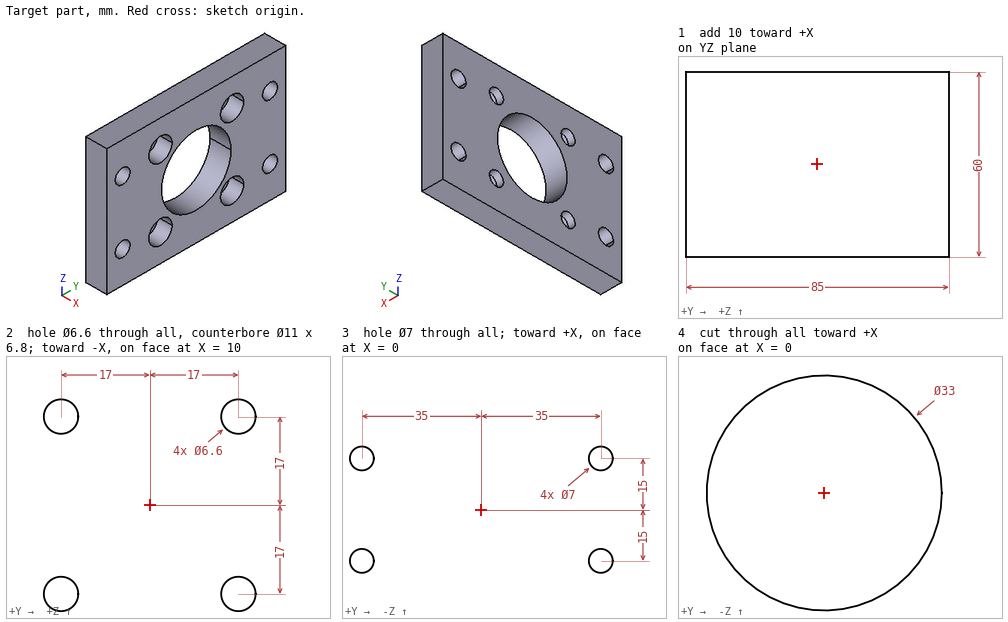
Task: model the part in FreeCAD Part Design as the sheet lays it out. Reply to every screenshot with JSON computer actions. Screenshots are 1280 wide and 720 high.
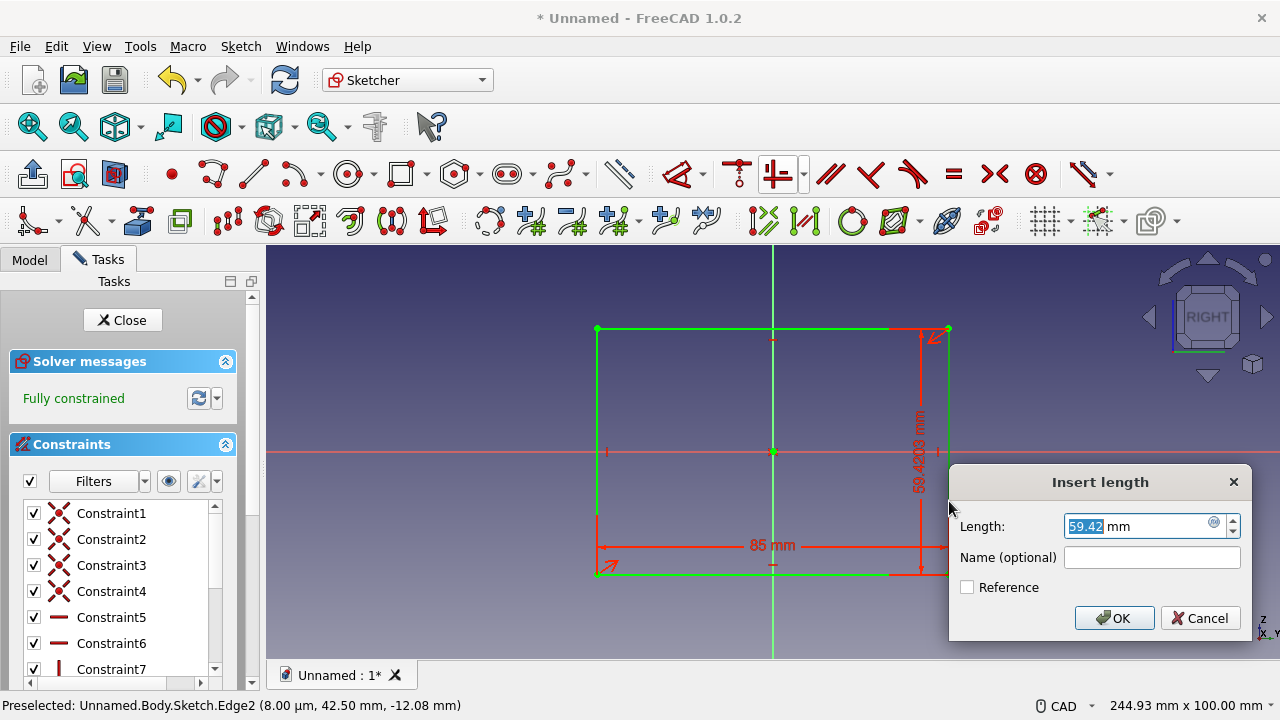
{"action": "type", "text": "60"}
{"action": "key", "text": "Return"}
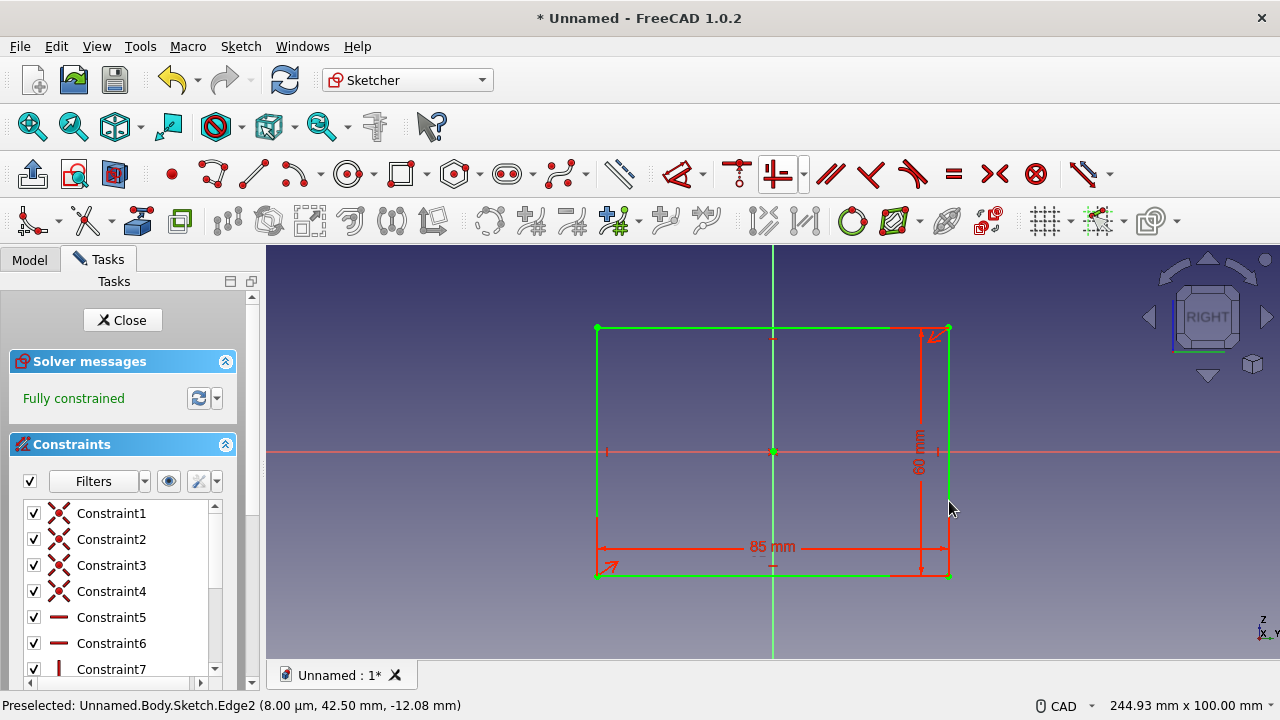
{"action": "left_click", "coordinate": [123, 320]}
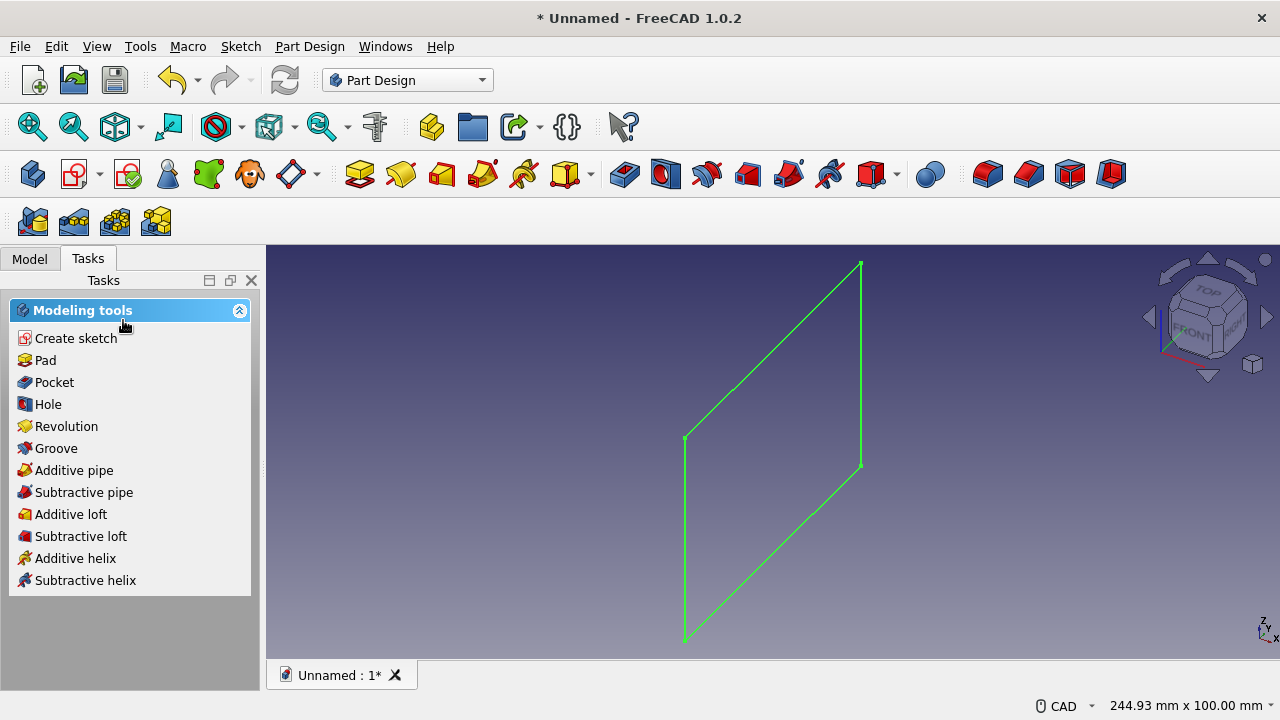
{"action": "left_click", "coordinate": [360, 174]}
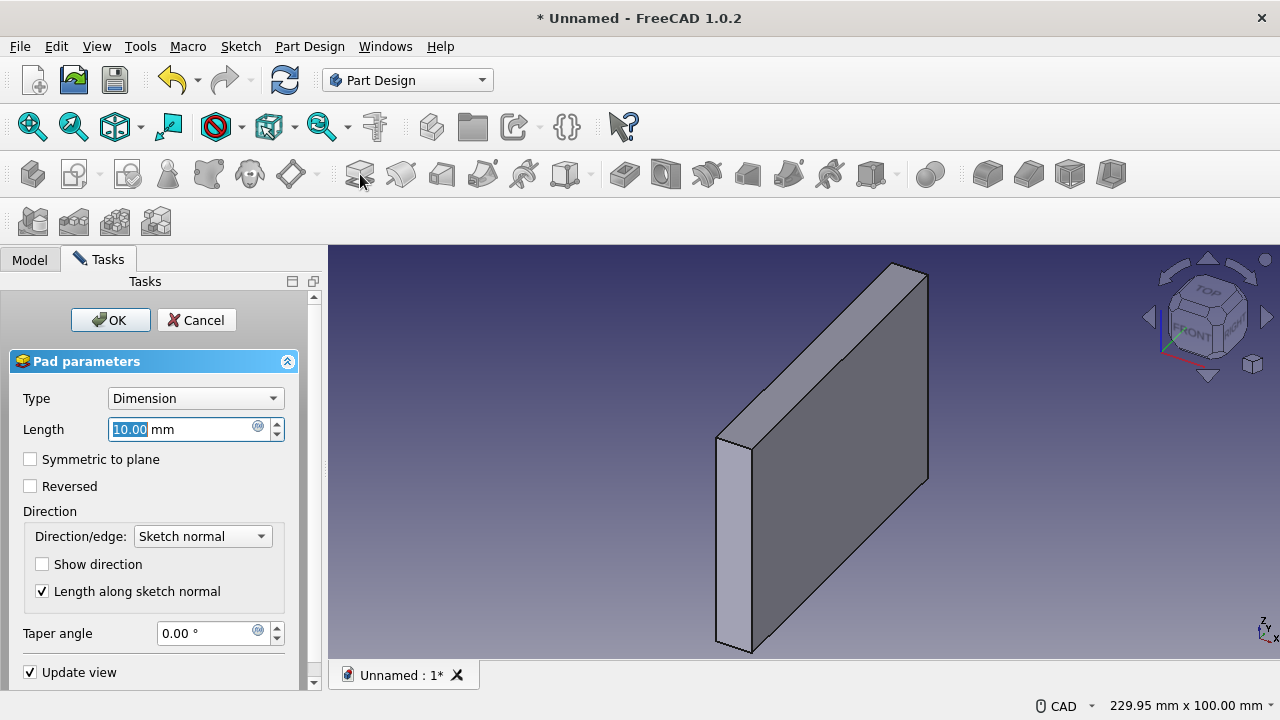
{"action": "type", "text": "10"}
{"action": "key", "text": "Tab"}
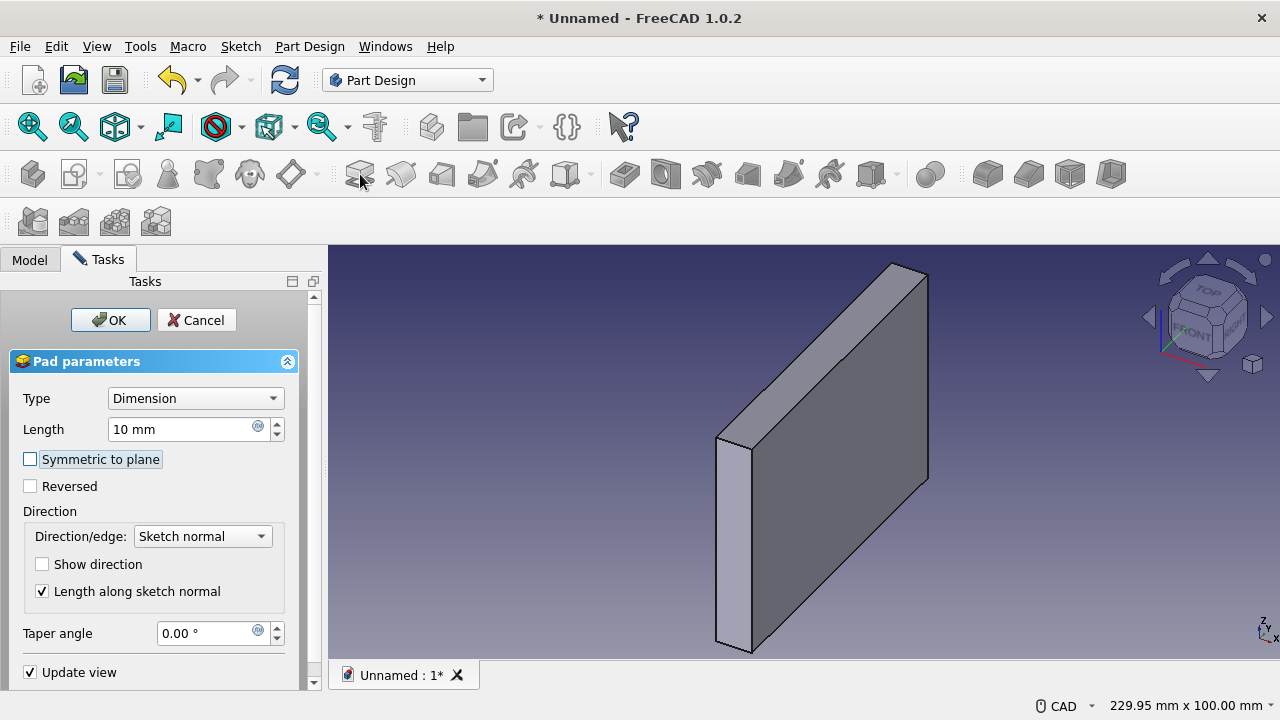
{"action": "left_click", "coordinate": [111, 320]}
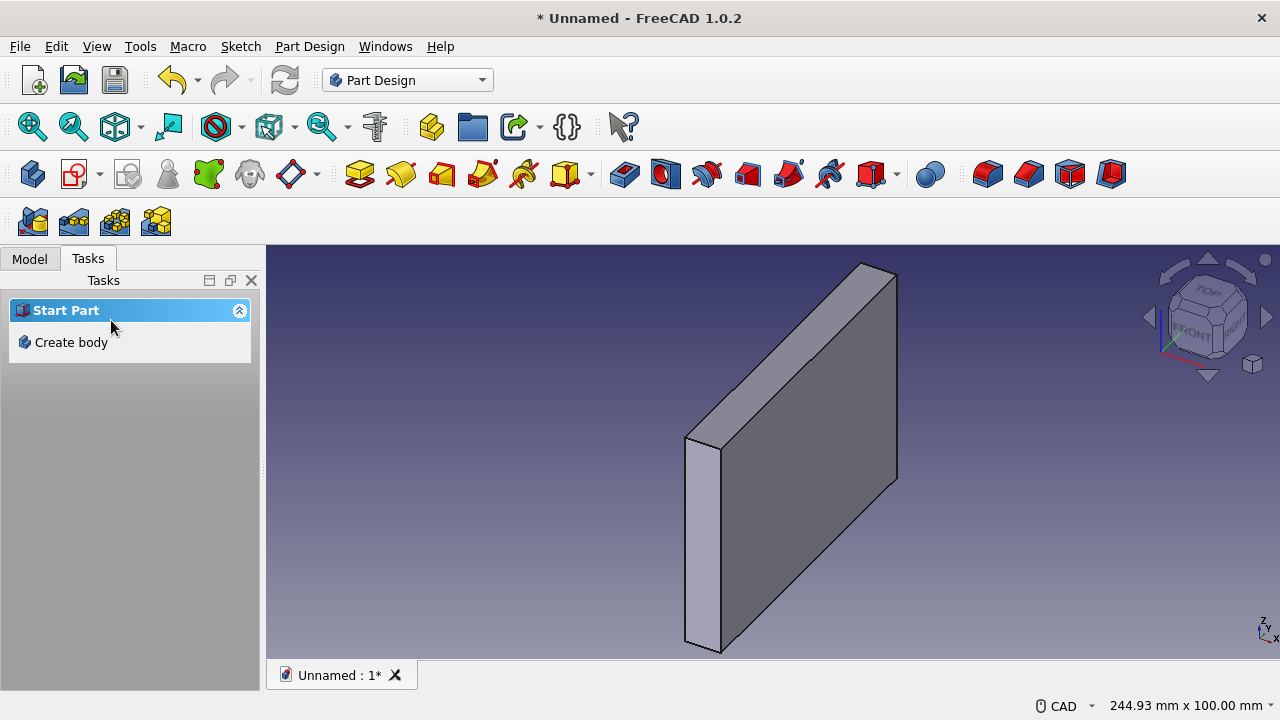
{"action": "left_click", "coordinate": [834, 438]}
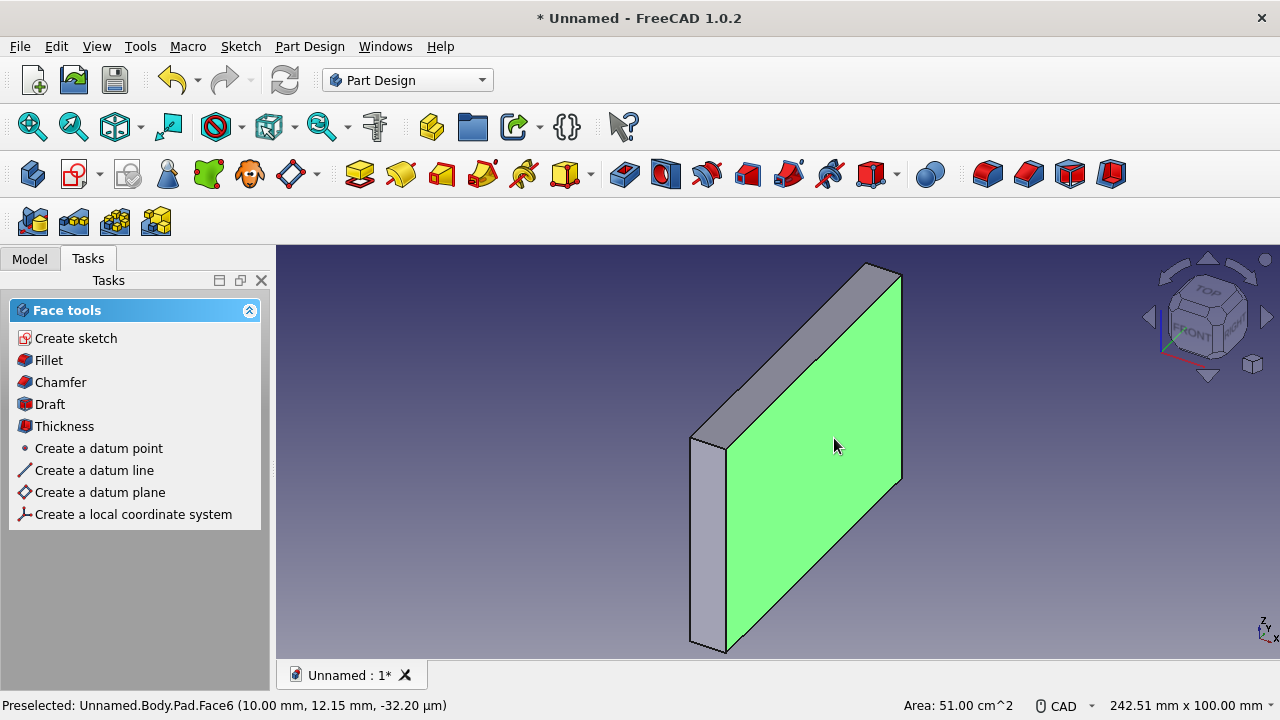
{"action": "left_click", "coordinate": [74, 174]}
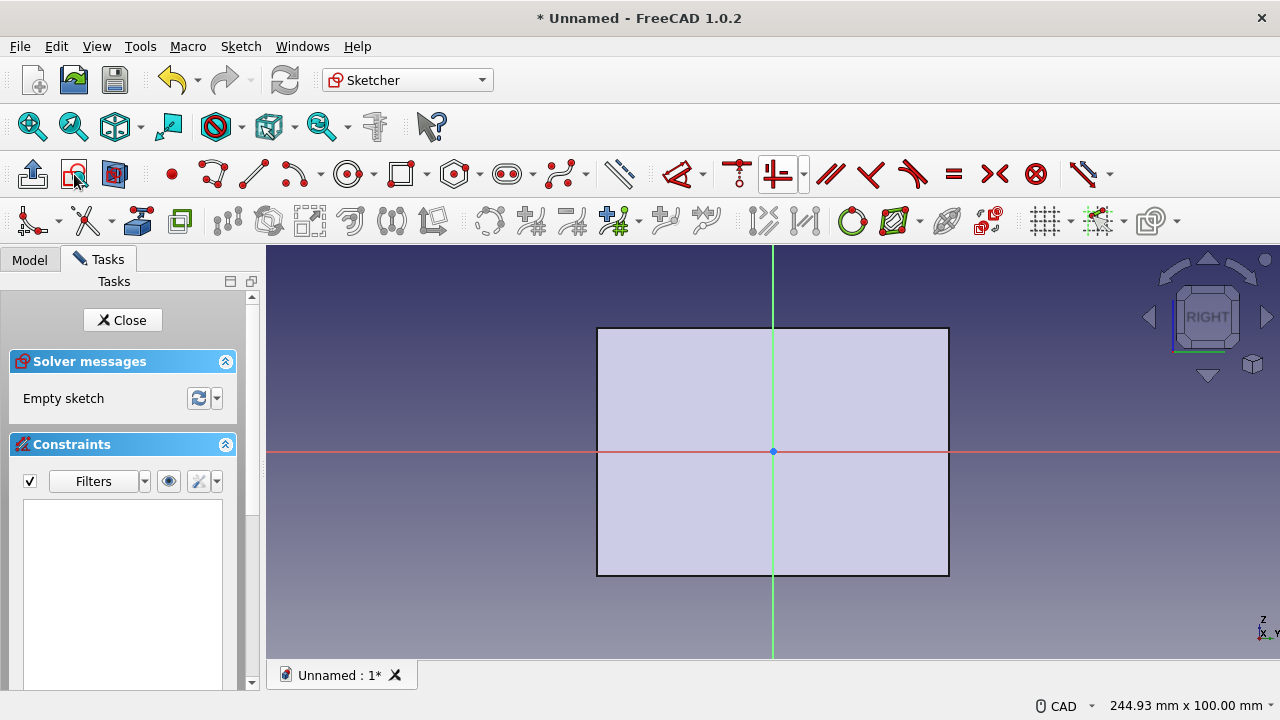
{"action": "scroll", "coordinate": [912, 452], "scroll_direction": "up", "scroll_amount": 2}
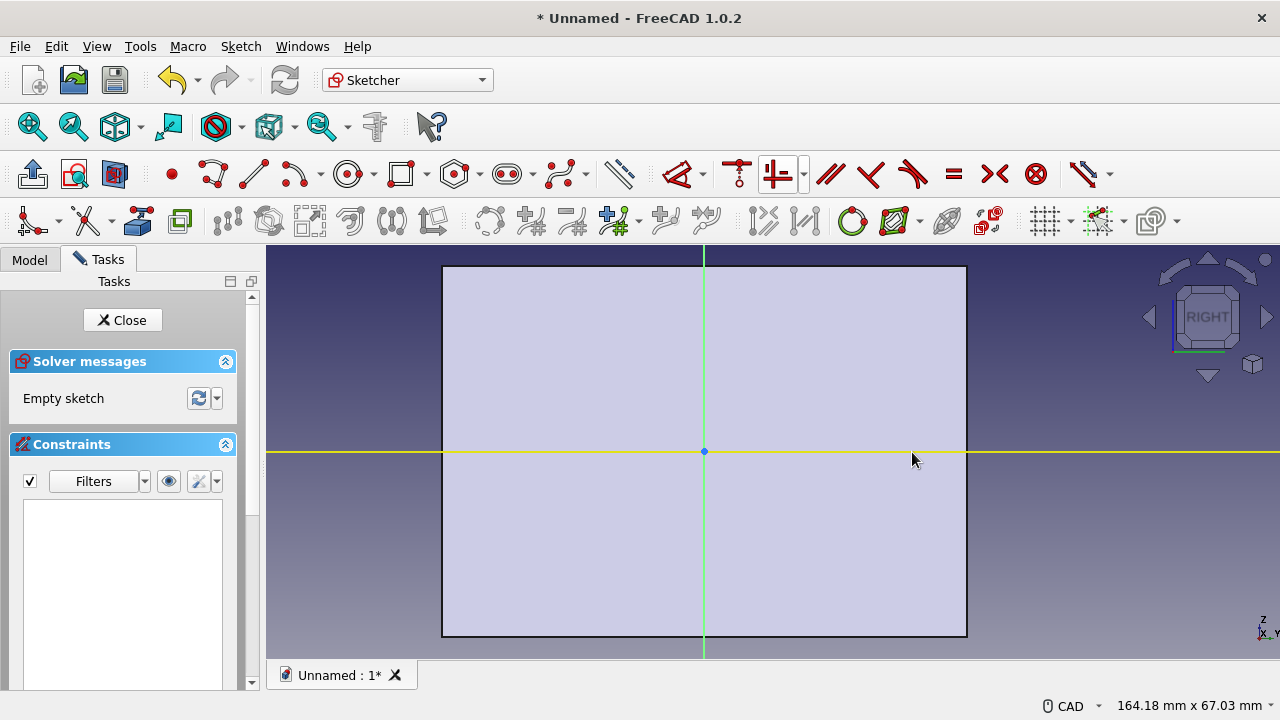
{"action": "key", "text": "g c"}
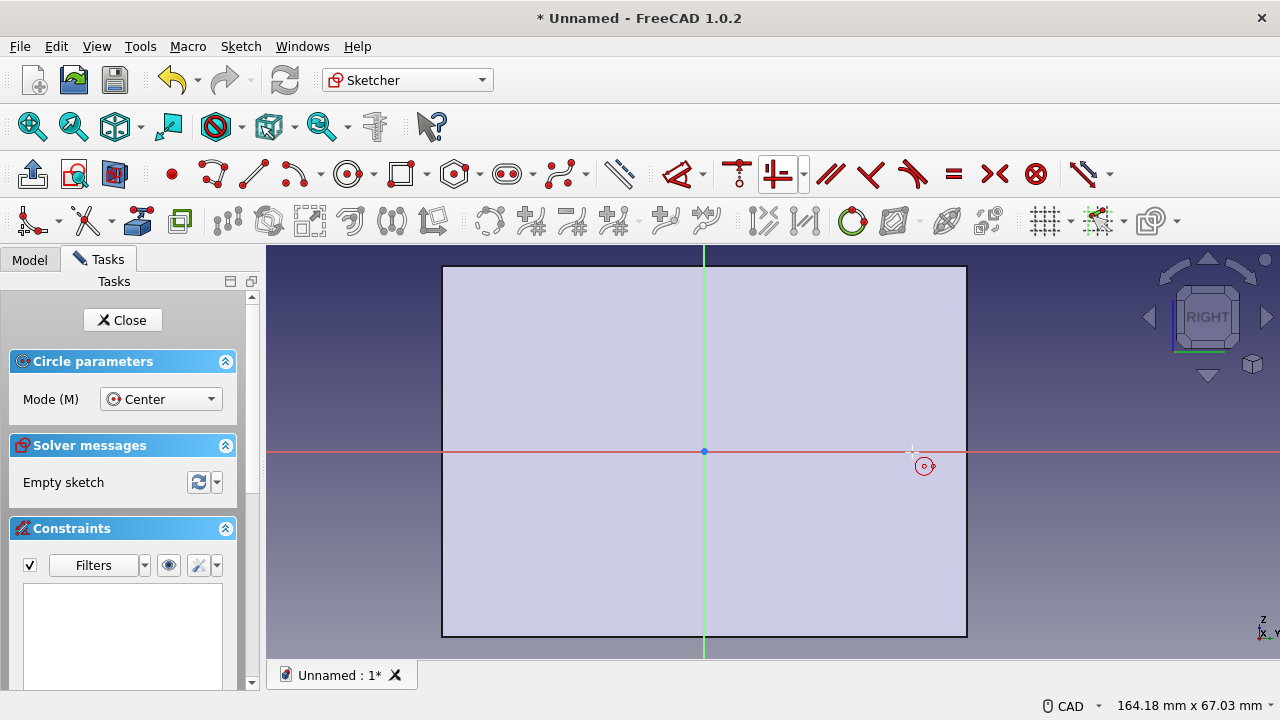
{"action": "left_click", "coordinate": [809, 347]}
{"action": "left_click", "coordinate": [824, 332]}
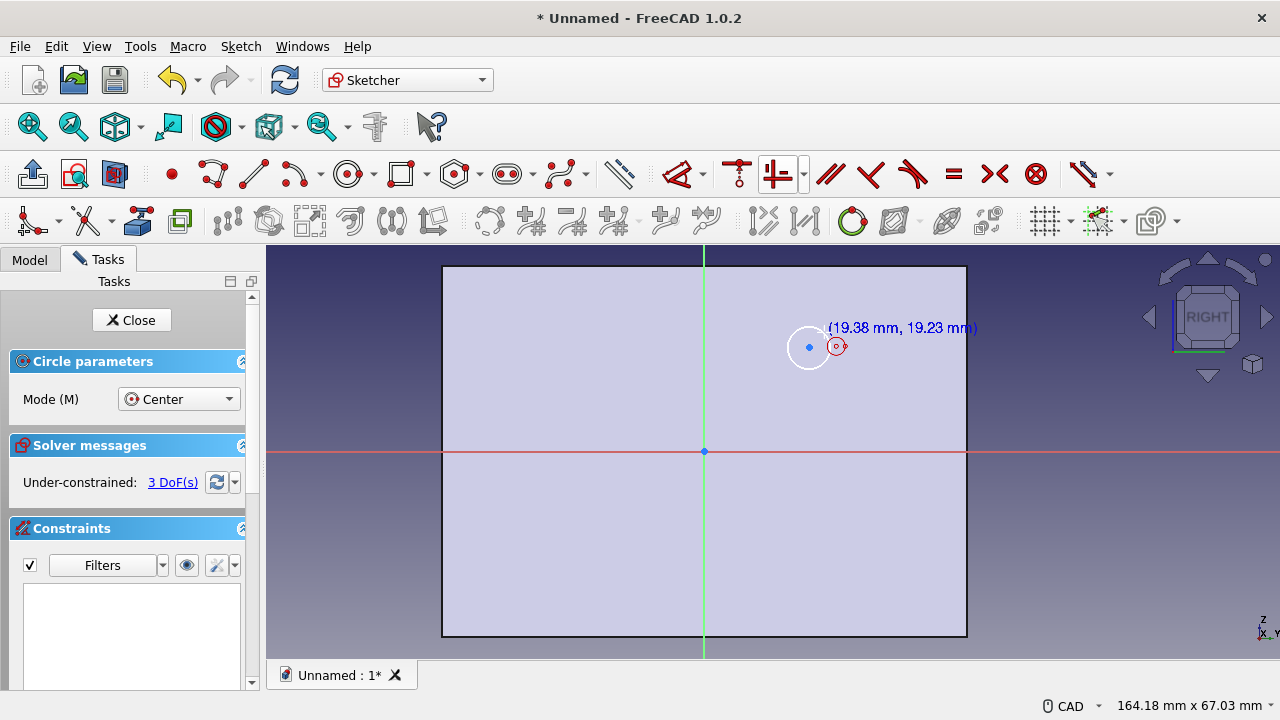
{"action": "left_click", "coordinate": [809, 557]}
{"action": "left_click", "coordinate": [824, 542]}